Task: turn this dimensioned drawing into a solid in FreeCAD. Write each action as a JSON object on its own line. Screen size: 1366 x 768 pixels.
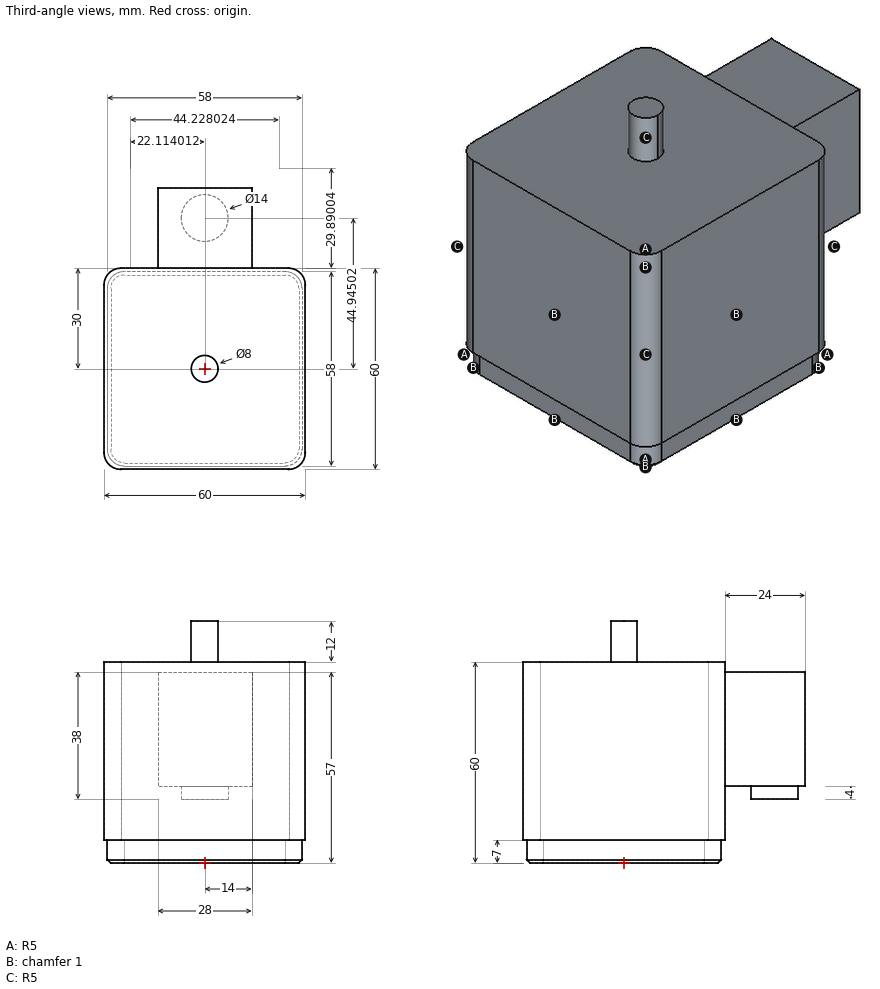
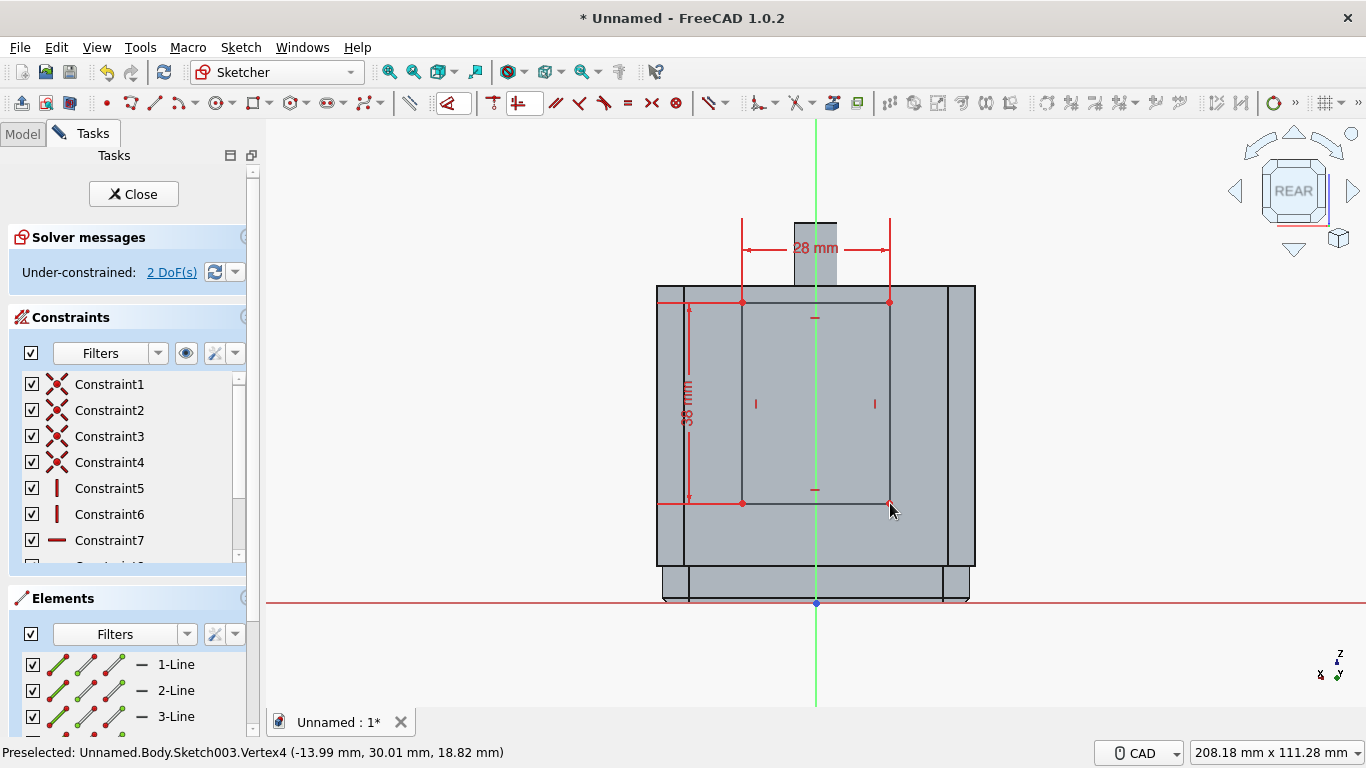
{"action": "left_click", "coordinate": [448, 104]}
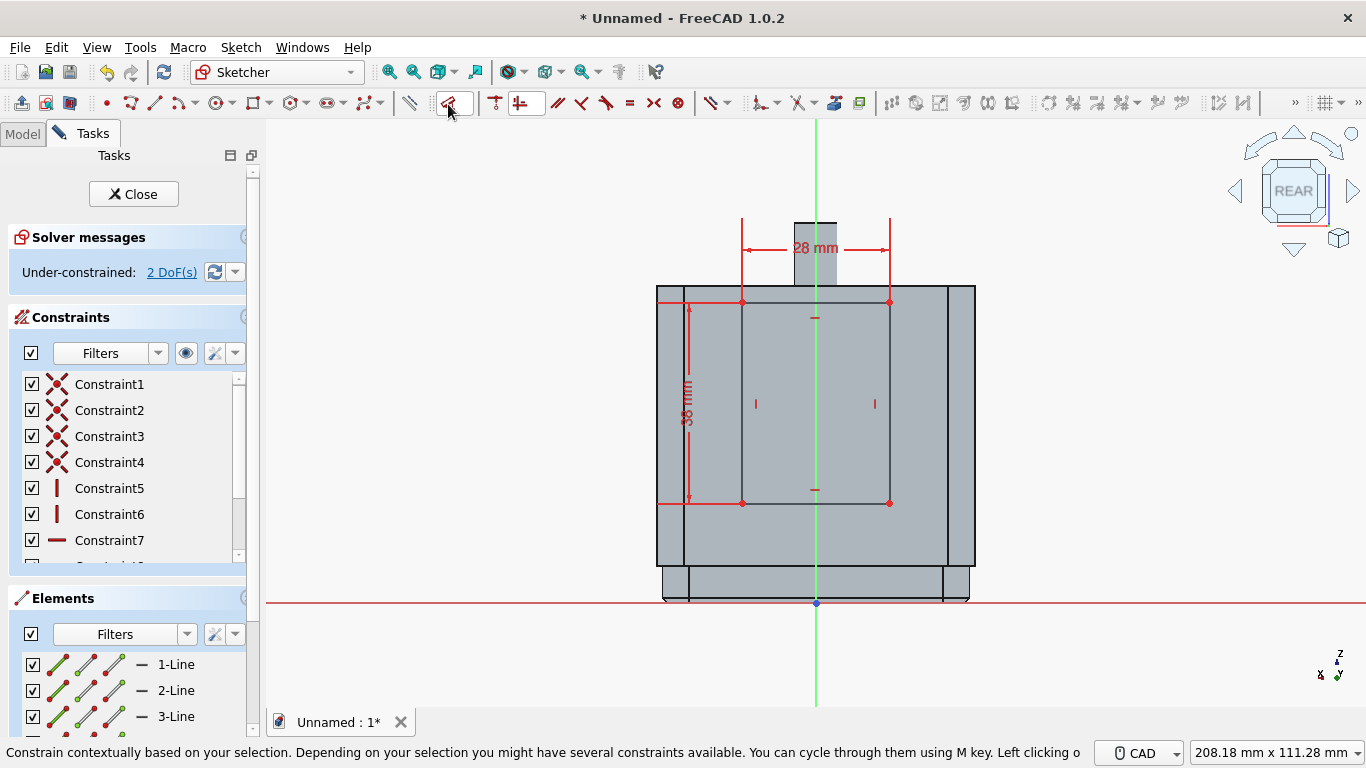
{"action": "left_click", "coordinate": [742, 303]}
{"action": "left_click", "coordinate": [779, 637]}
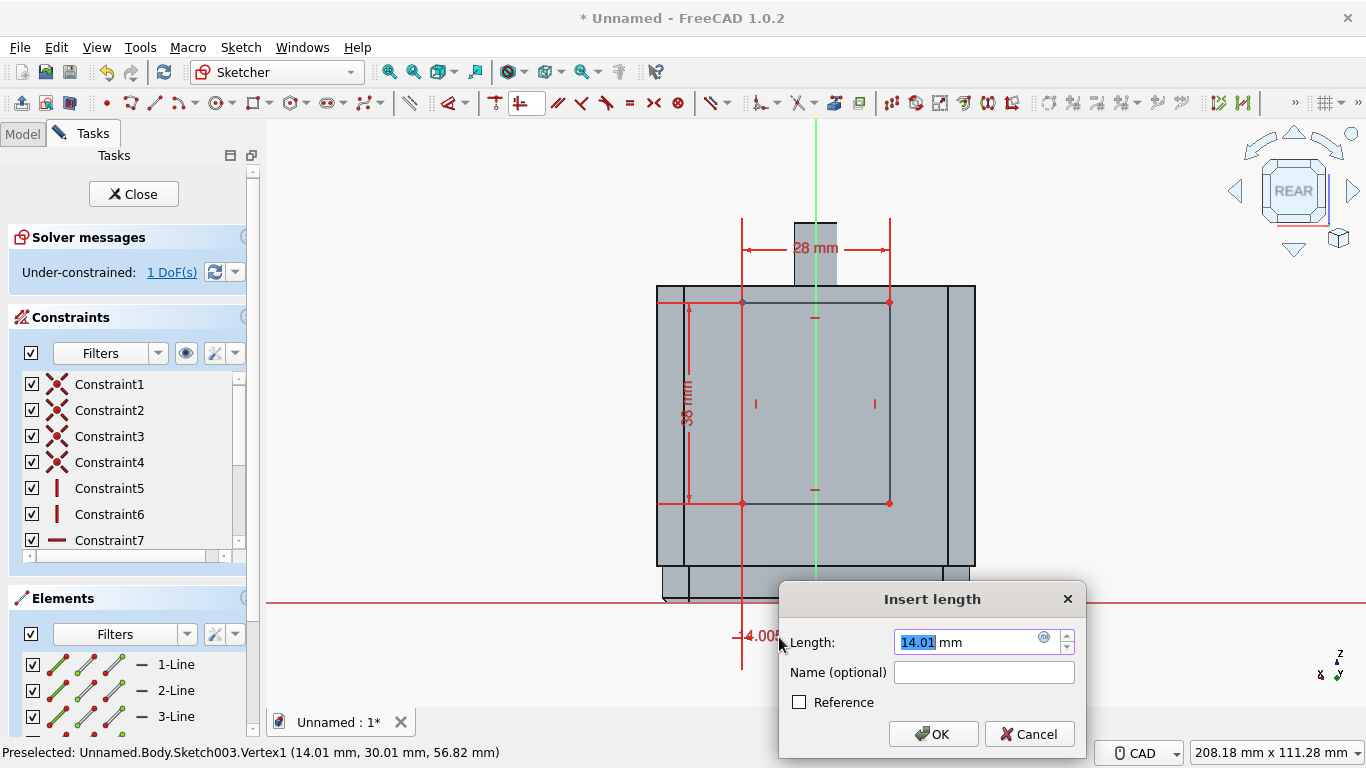
{"action": "type", "text": "14"}
{"action": "key", "text": "Return"}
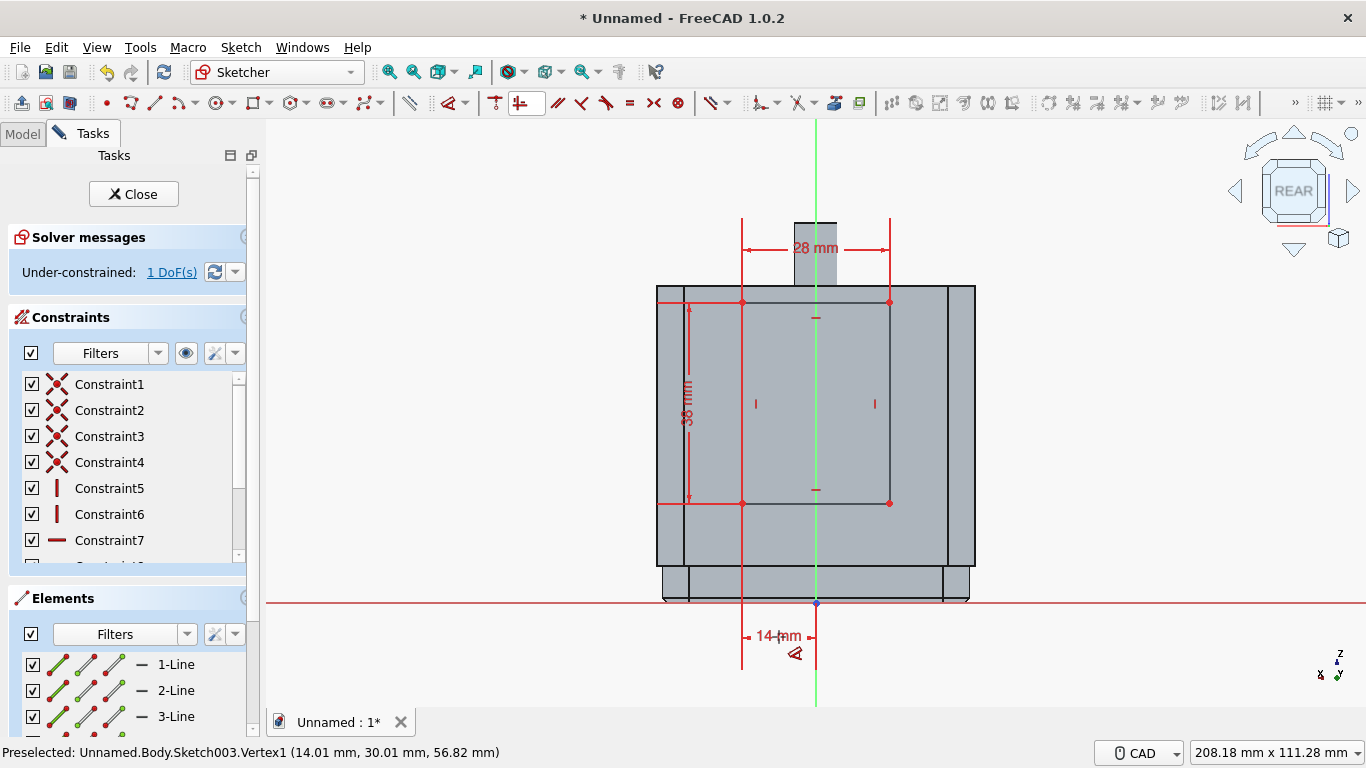
{"action": "left_click", "coordinate": [742, 303]}
{"action": "left_click", "coordinate": [708, 453]}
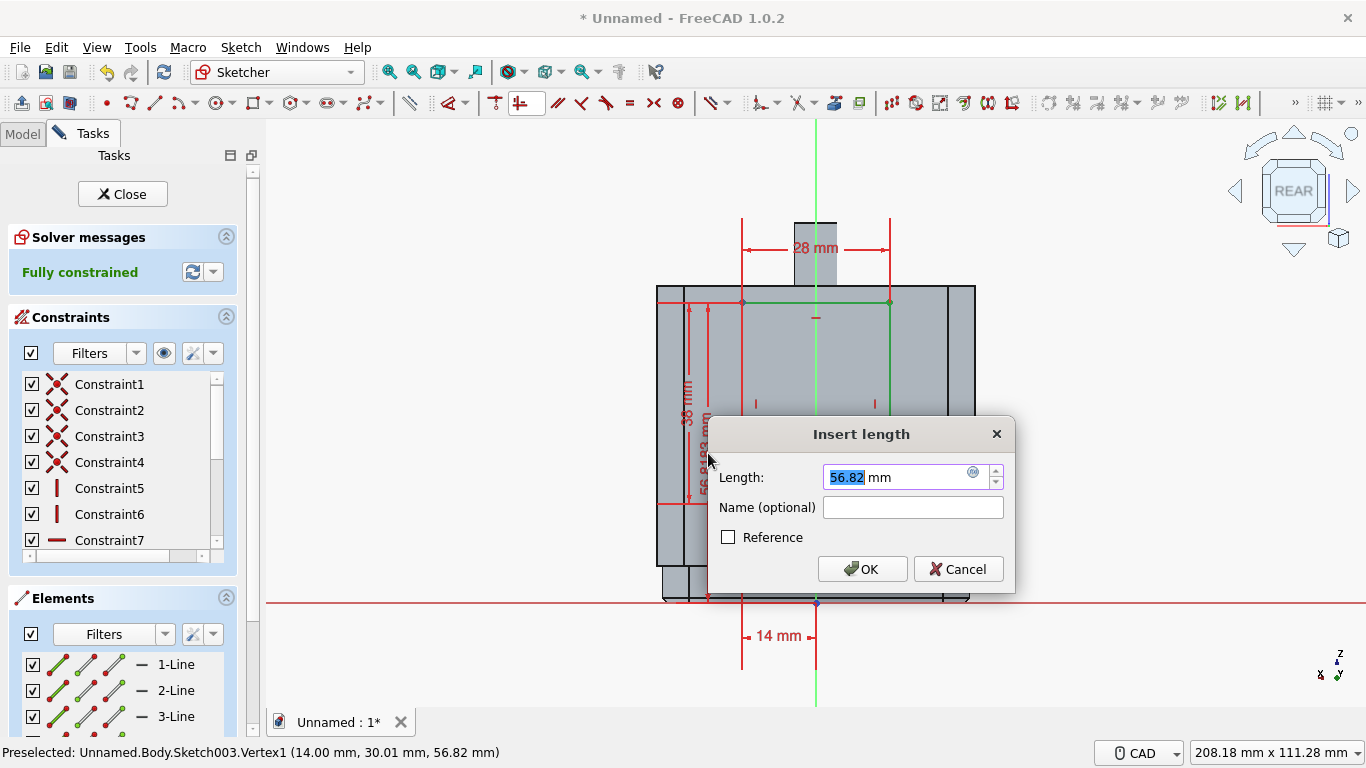
{"action": "type", "text": "57"}
{"action": "key", "text": "Return"}
{"action": "key", "text": "Escape"}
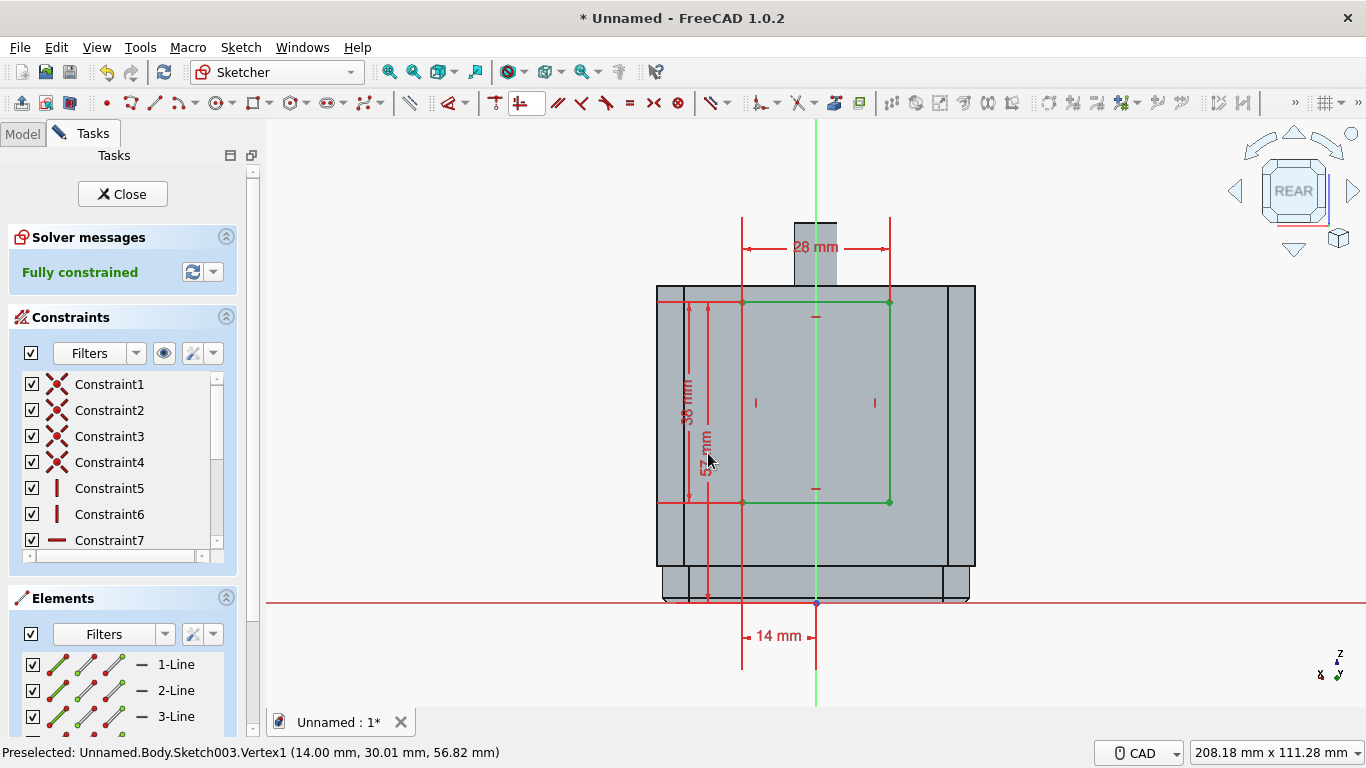
{"action": "left_click", "coordinate": [123, 194]}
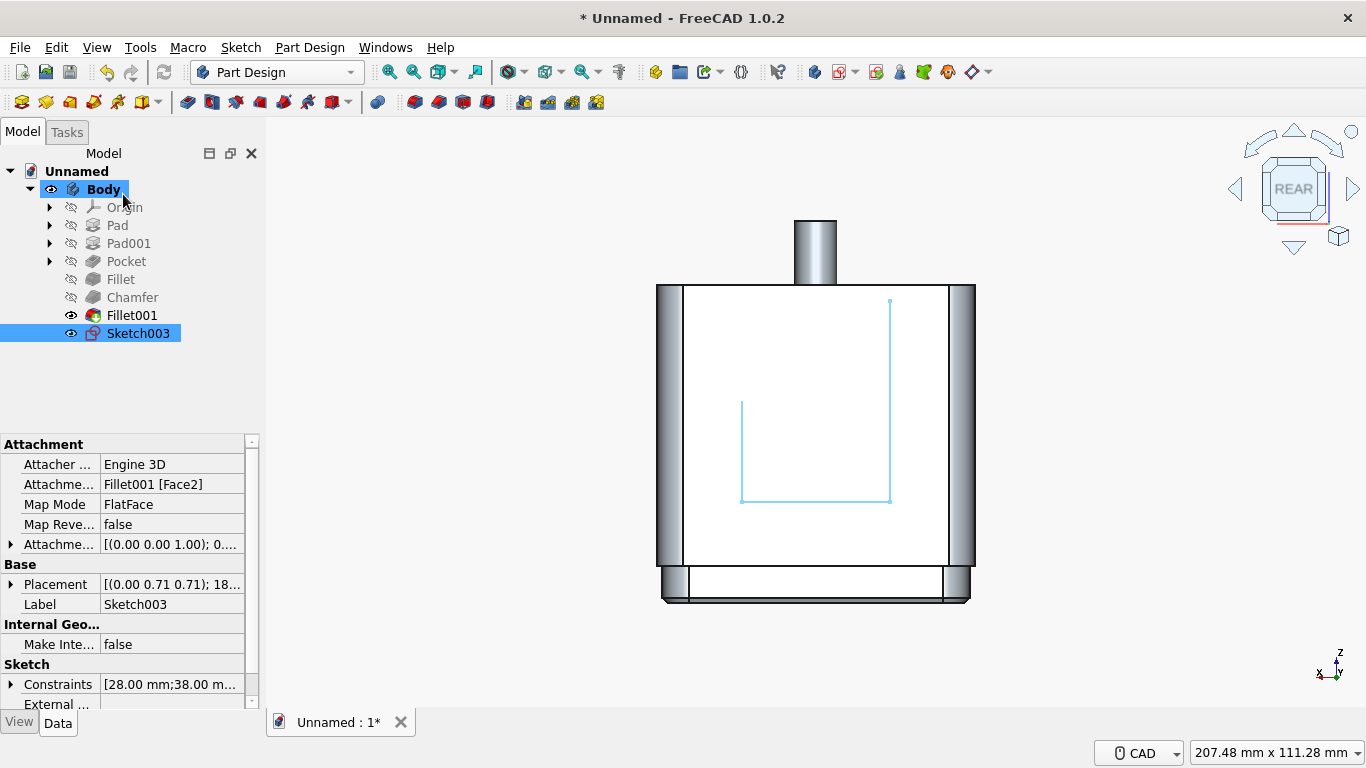
{"action": "left_click", "coordinate": [22, 102]}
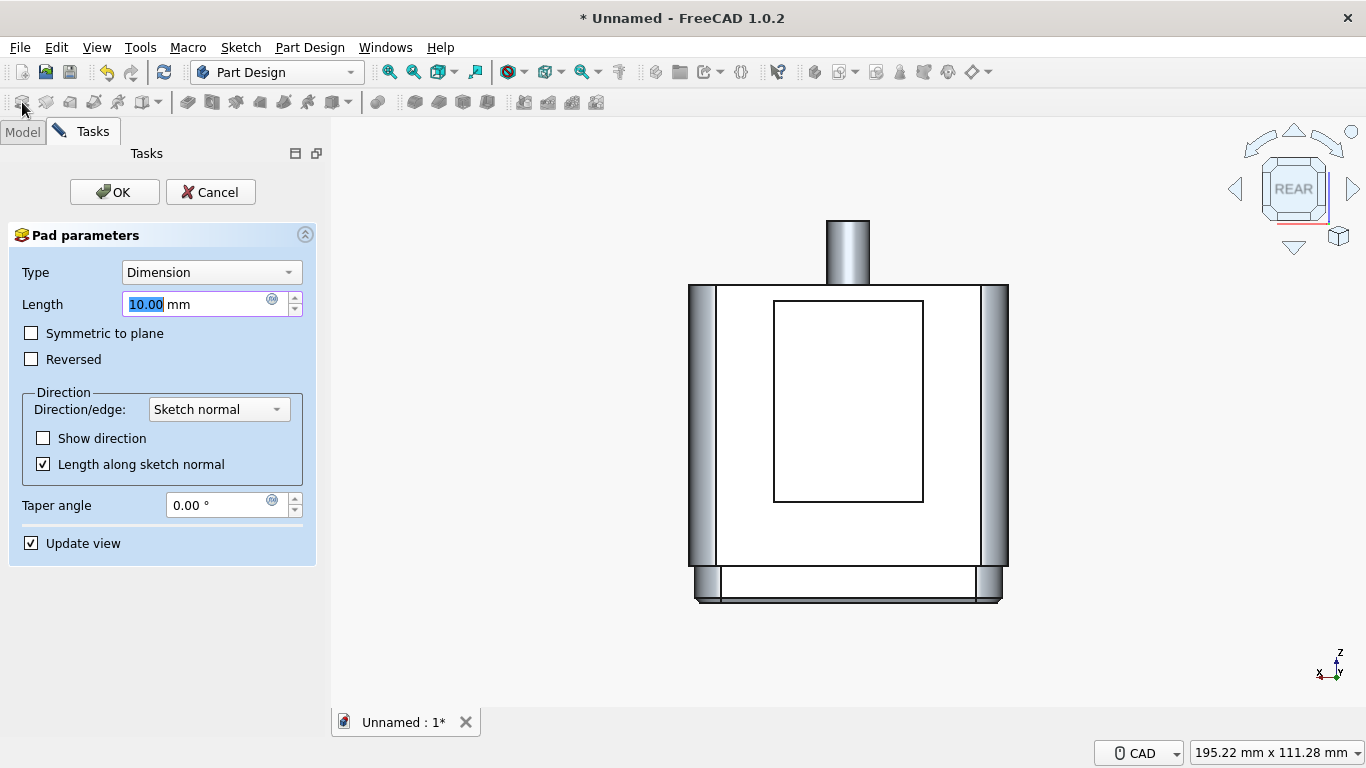
{"action": "type", "text": "24"}
{"action": "key", "text": "Tab"}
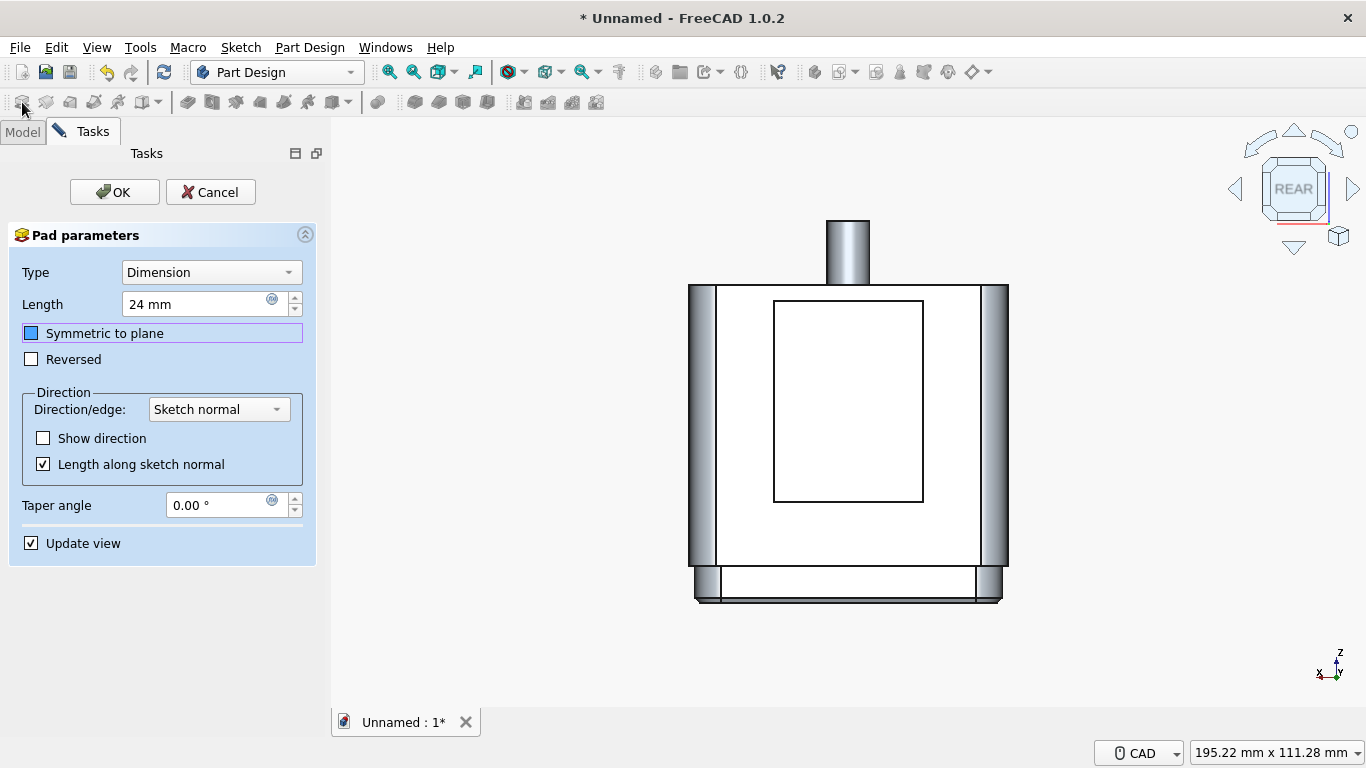
{"action": "left_click", "coordinate": [115, 192]}